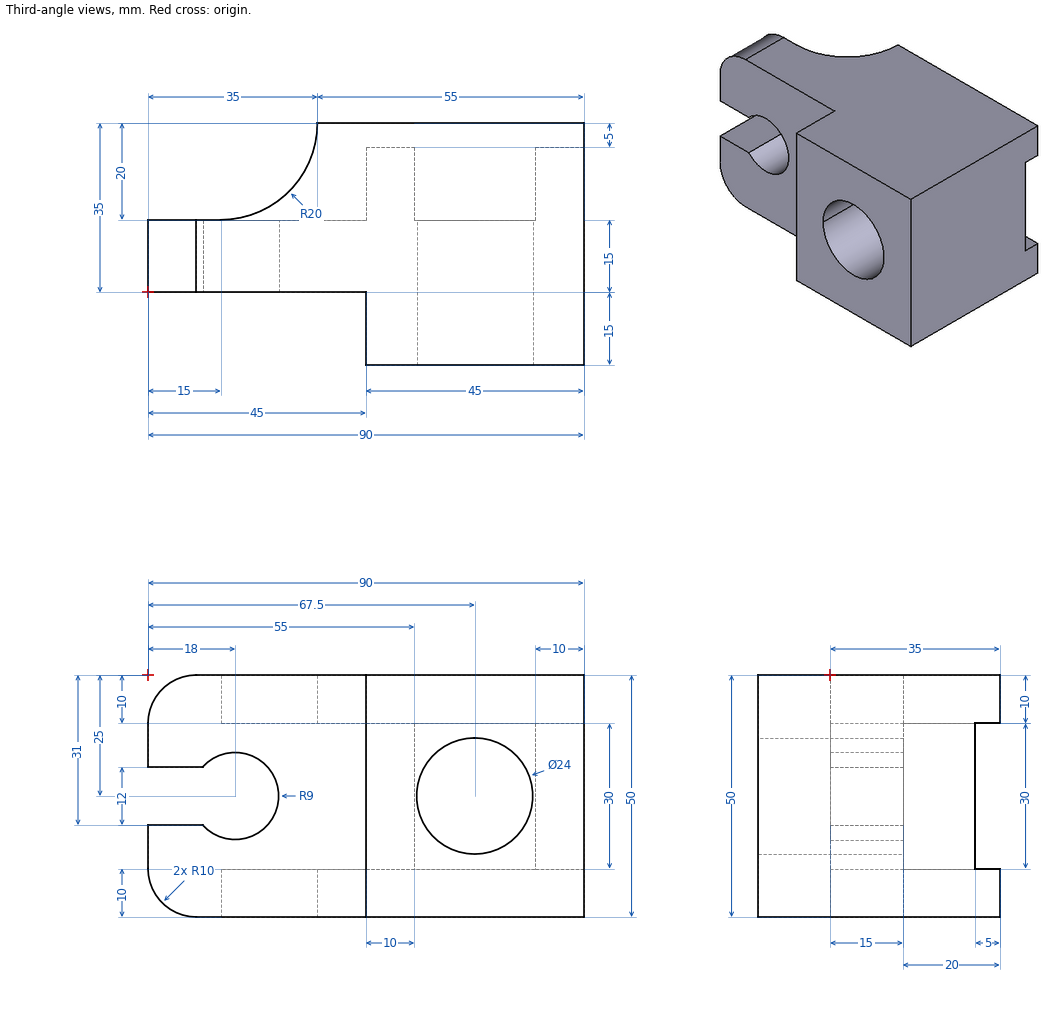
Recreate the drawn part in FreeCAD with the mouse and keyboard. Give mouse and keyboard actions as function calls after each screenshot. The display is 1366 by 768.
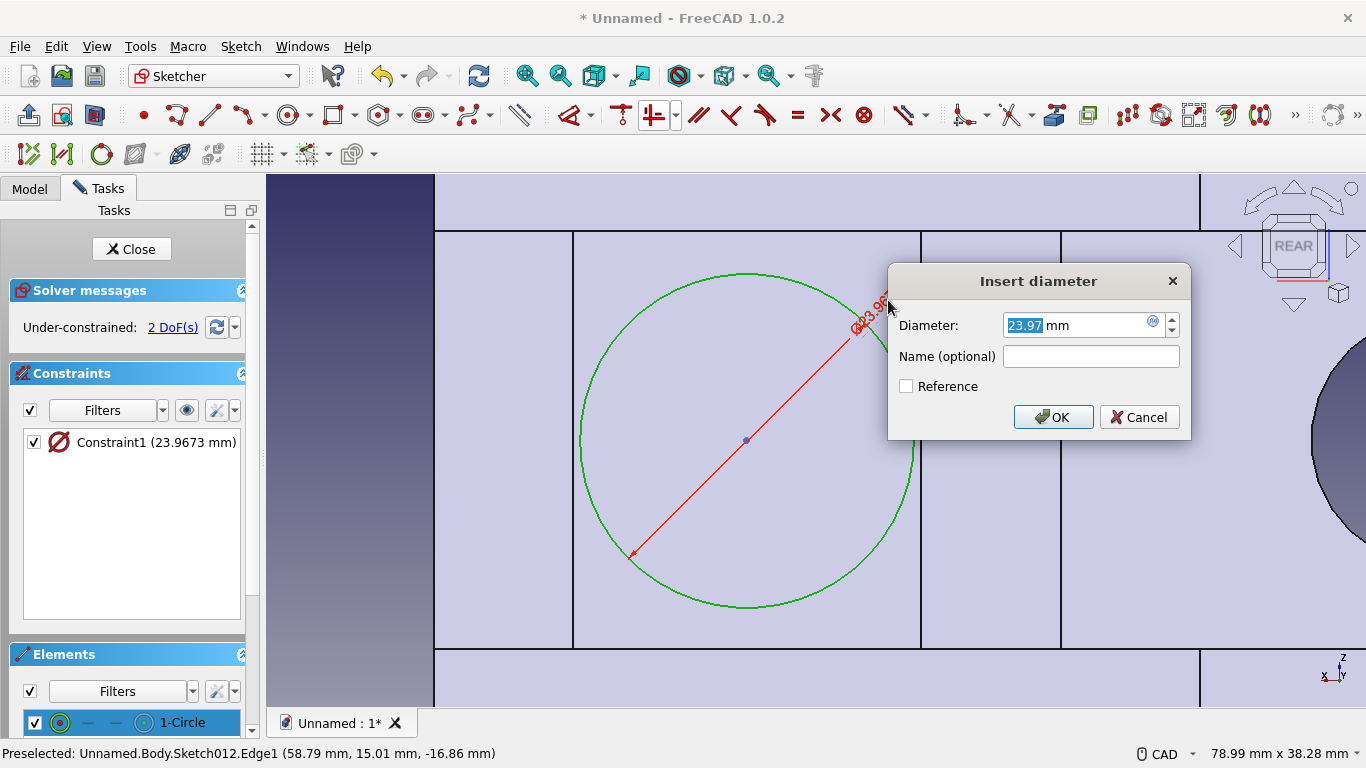
text(24)
key(Return)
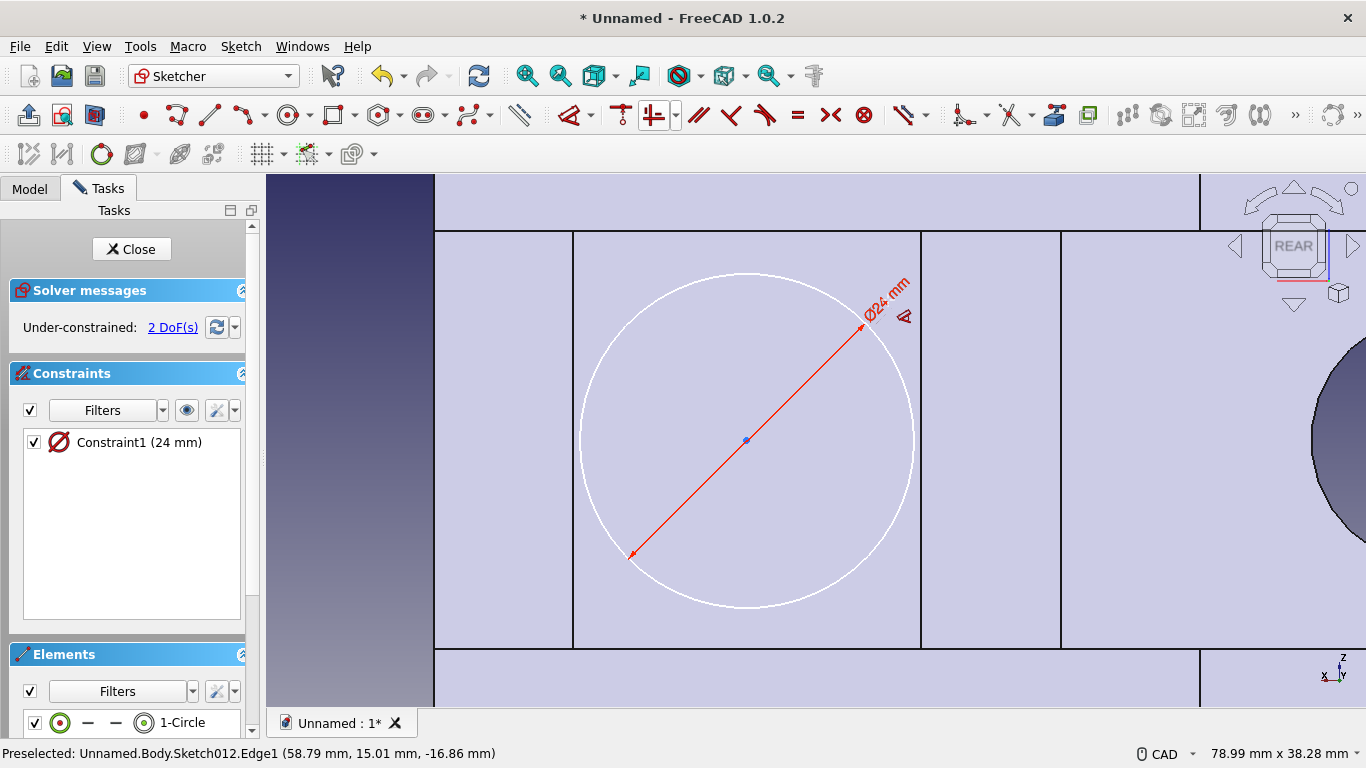
click(747, 441)
click(713, 321)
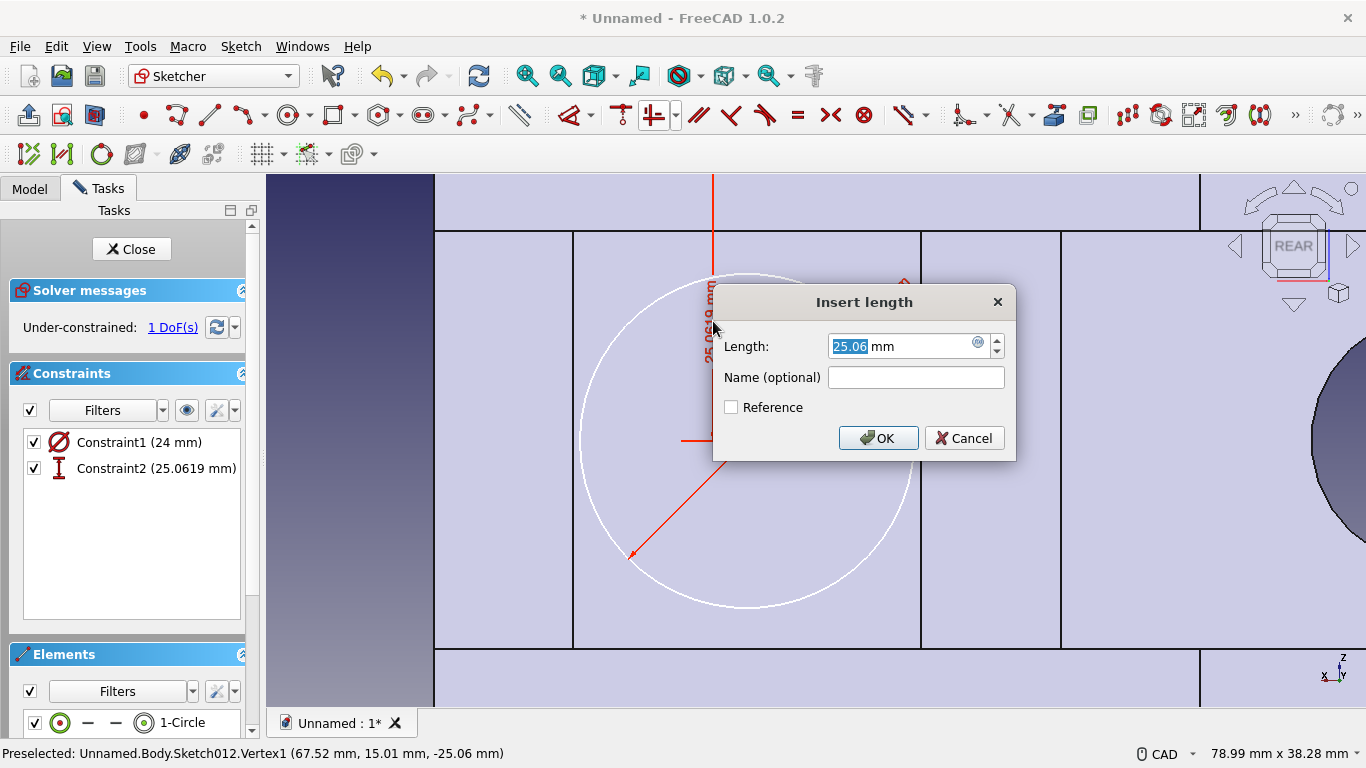
text(25)
key(Return)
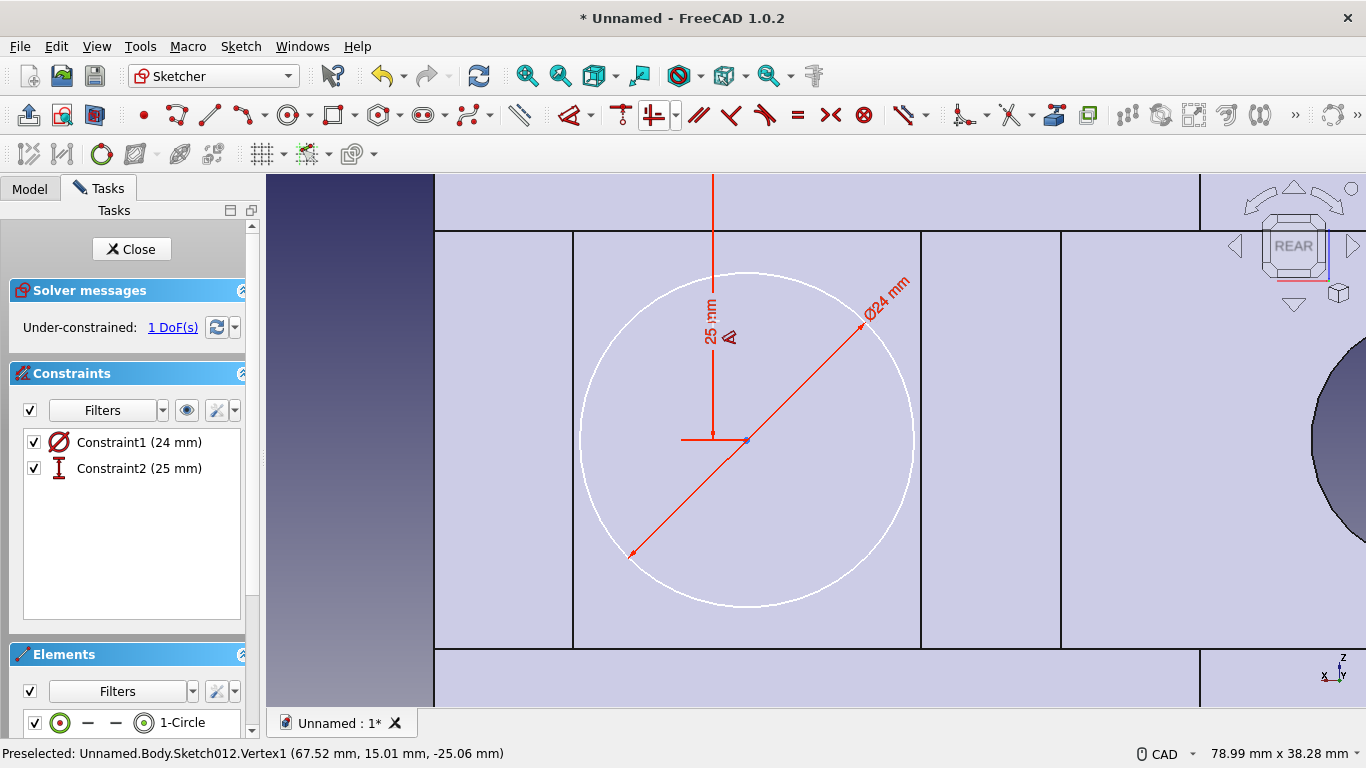
click(747, 440)
click(974, 474)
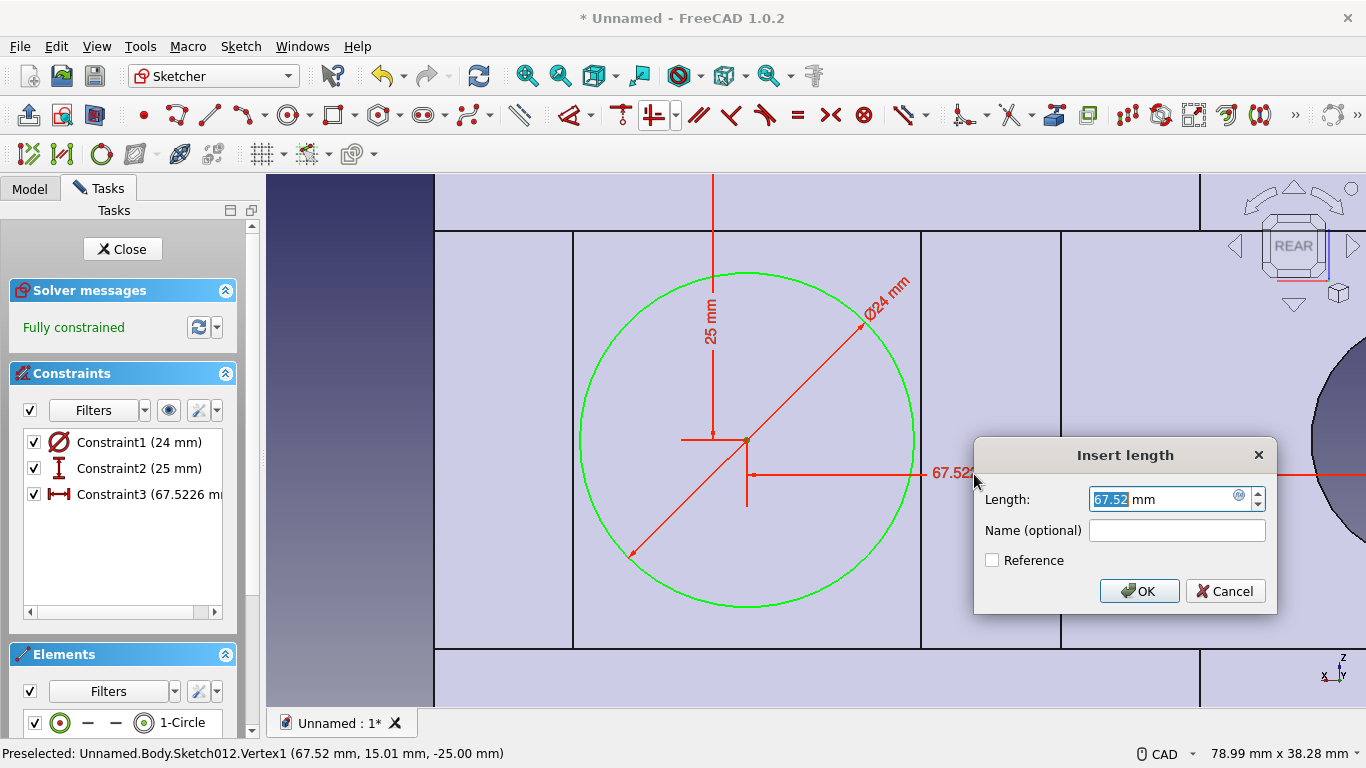
text(67.5)
key(Return)
key(Escape)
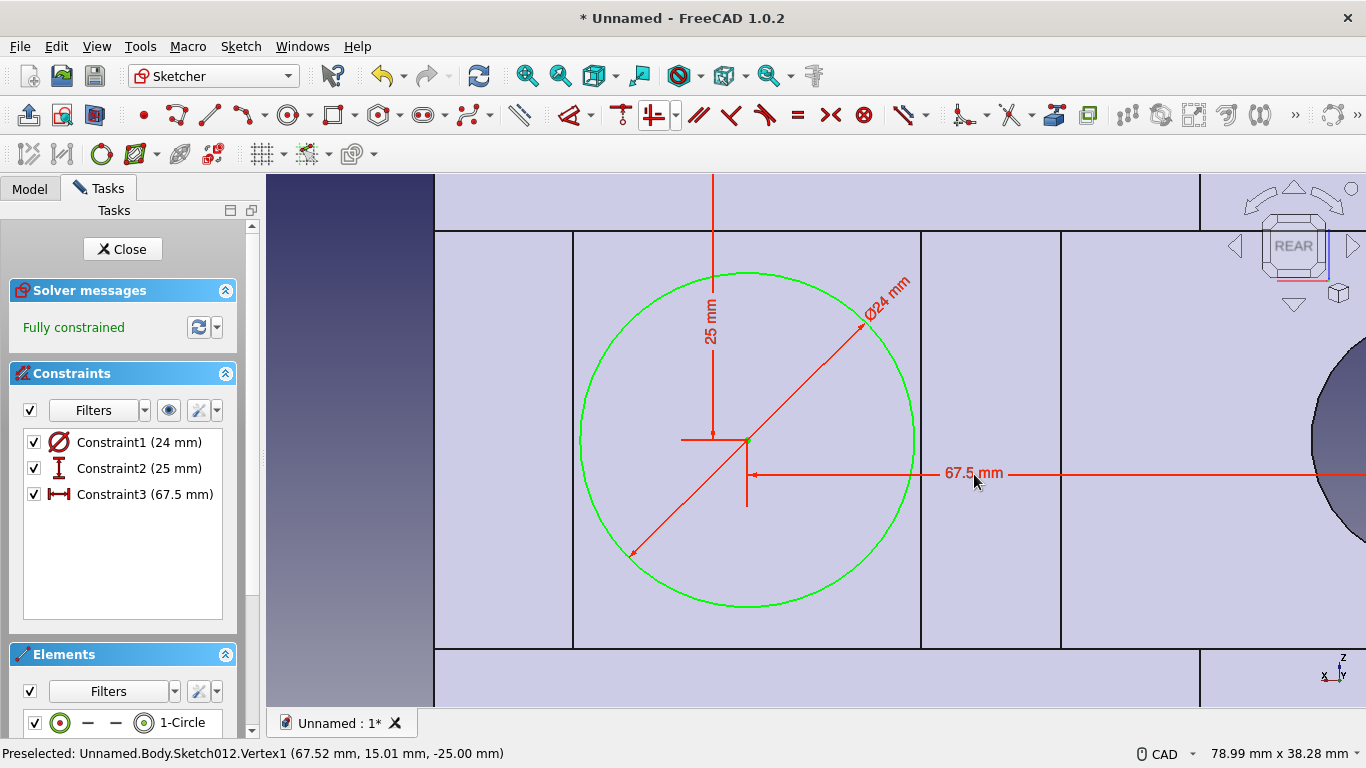
click(123, 249)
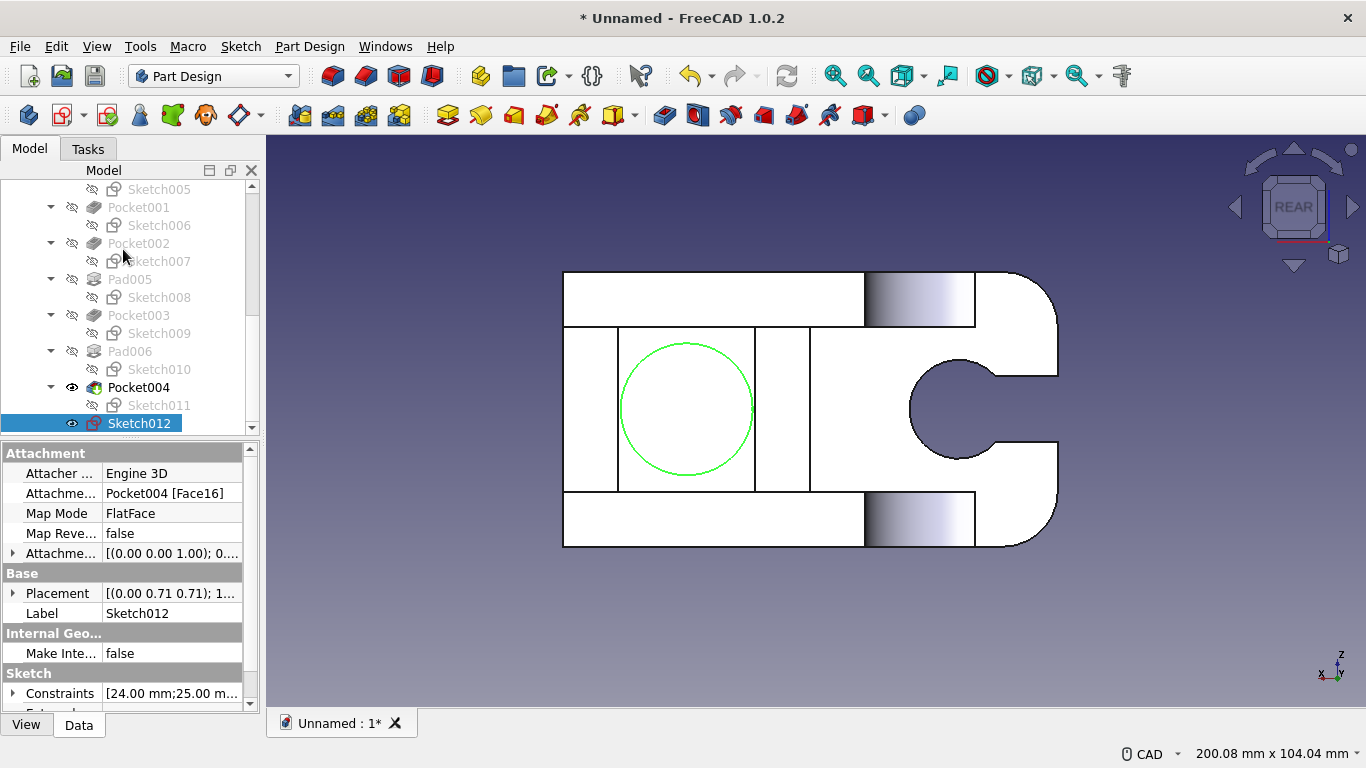
click(665, 116)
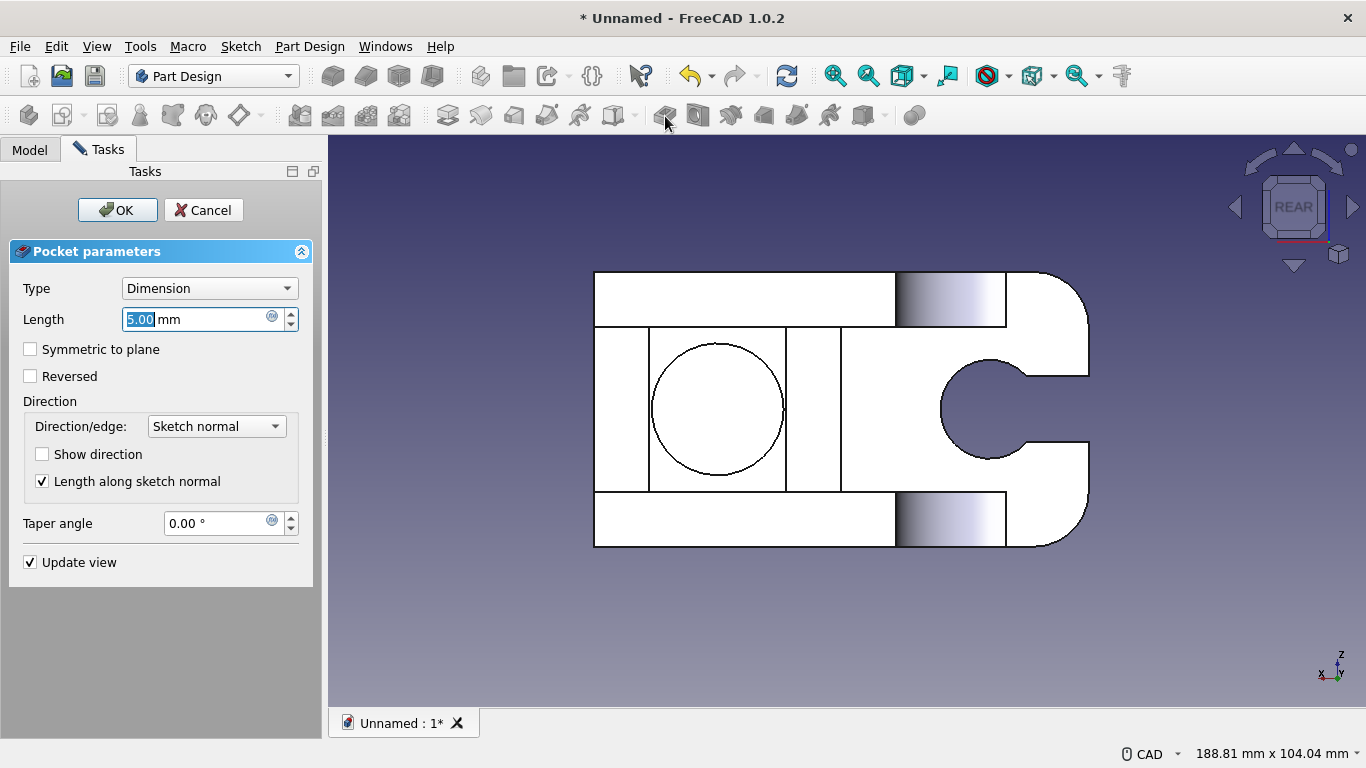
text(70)
key(Tab)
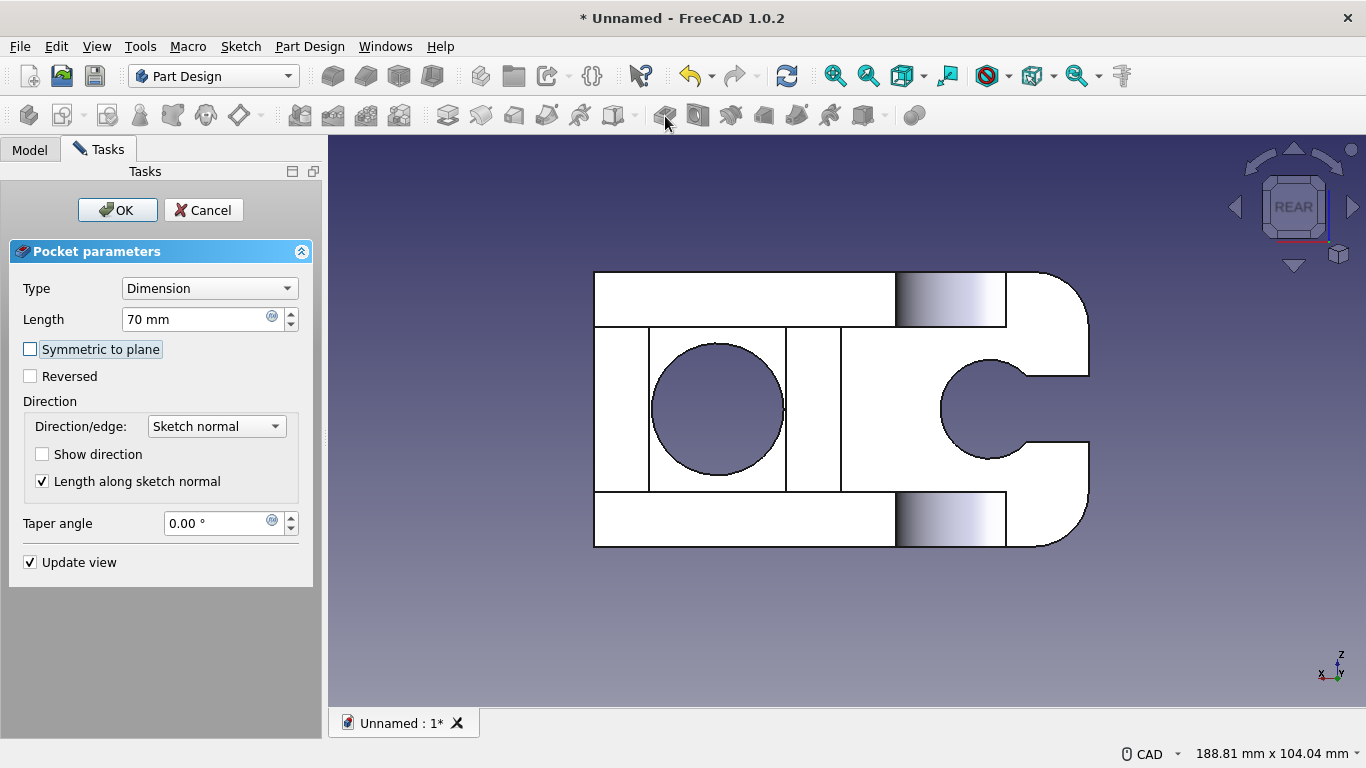
click(118, 210)